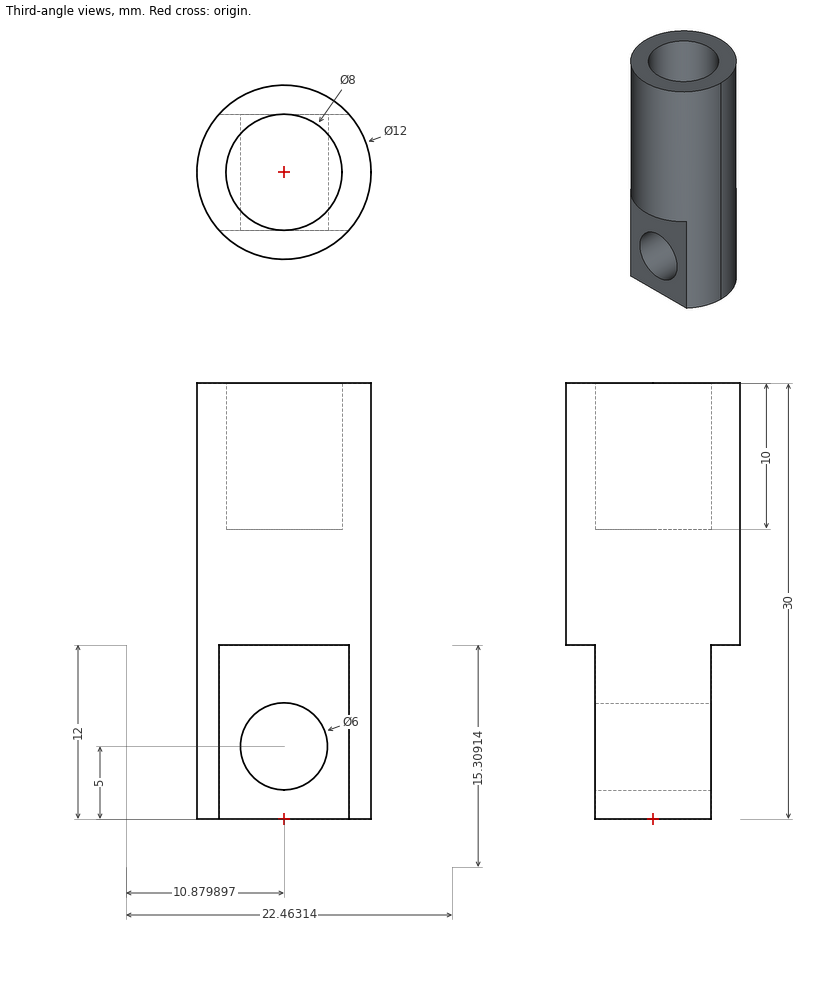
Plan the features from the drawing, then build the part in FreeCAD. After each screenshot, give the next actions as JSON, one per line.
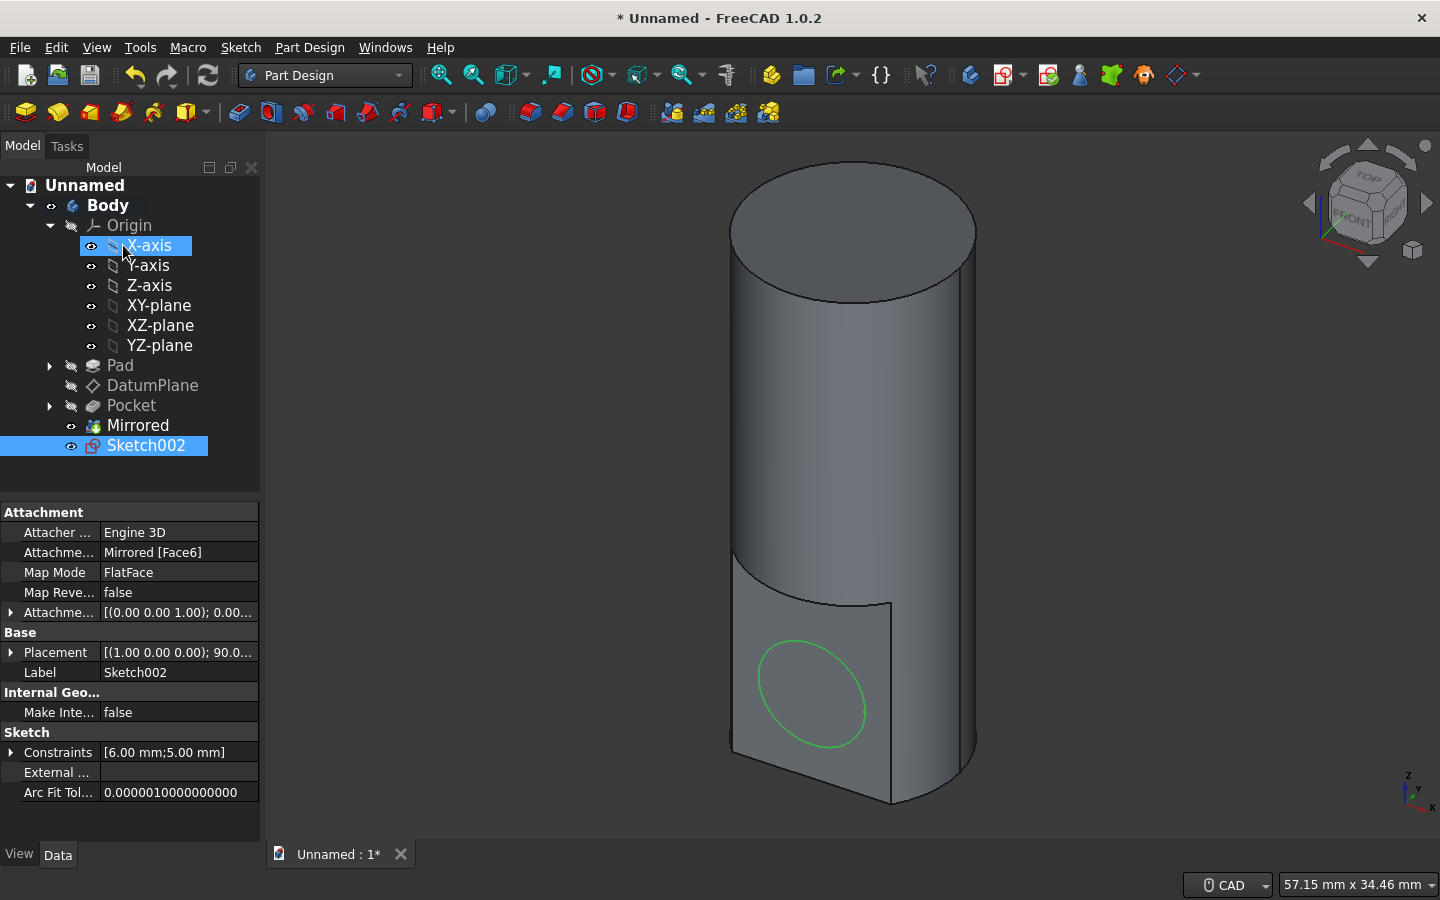
{"action": "left_click", "coordinate": [240, 112]}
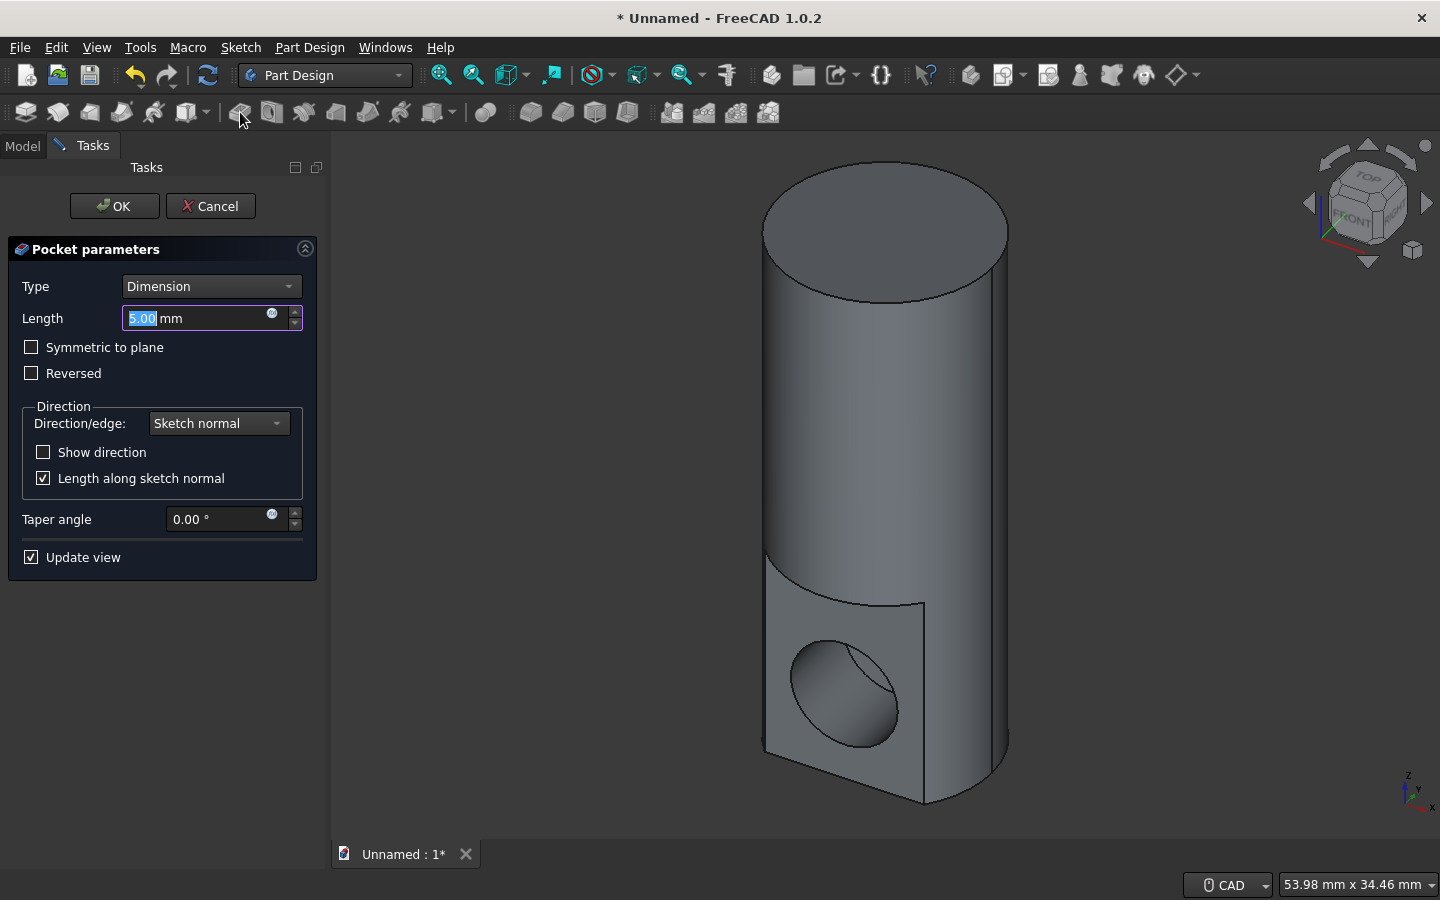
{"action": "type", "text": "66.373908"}
{"action": "key", "text": "Tab"}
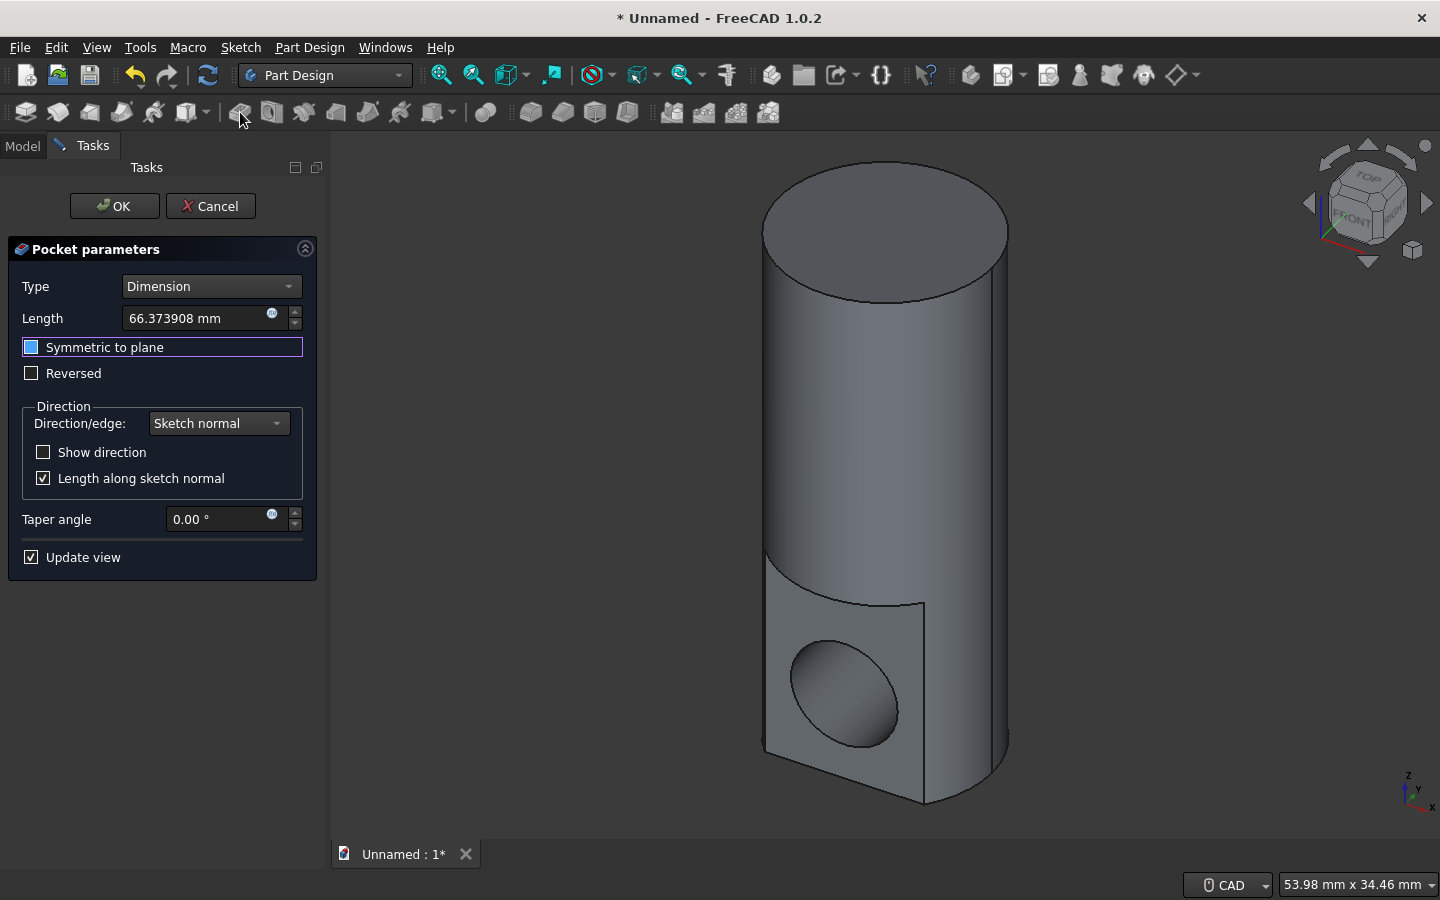
{"action": "left_click", "coordinate": [30, 347]}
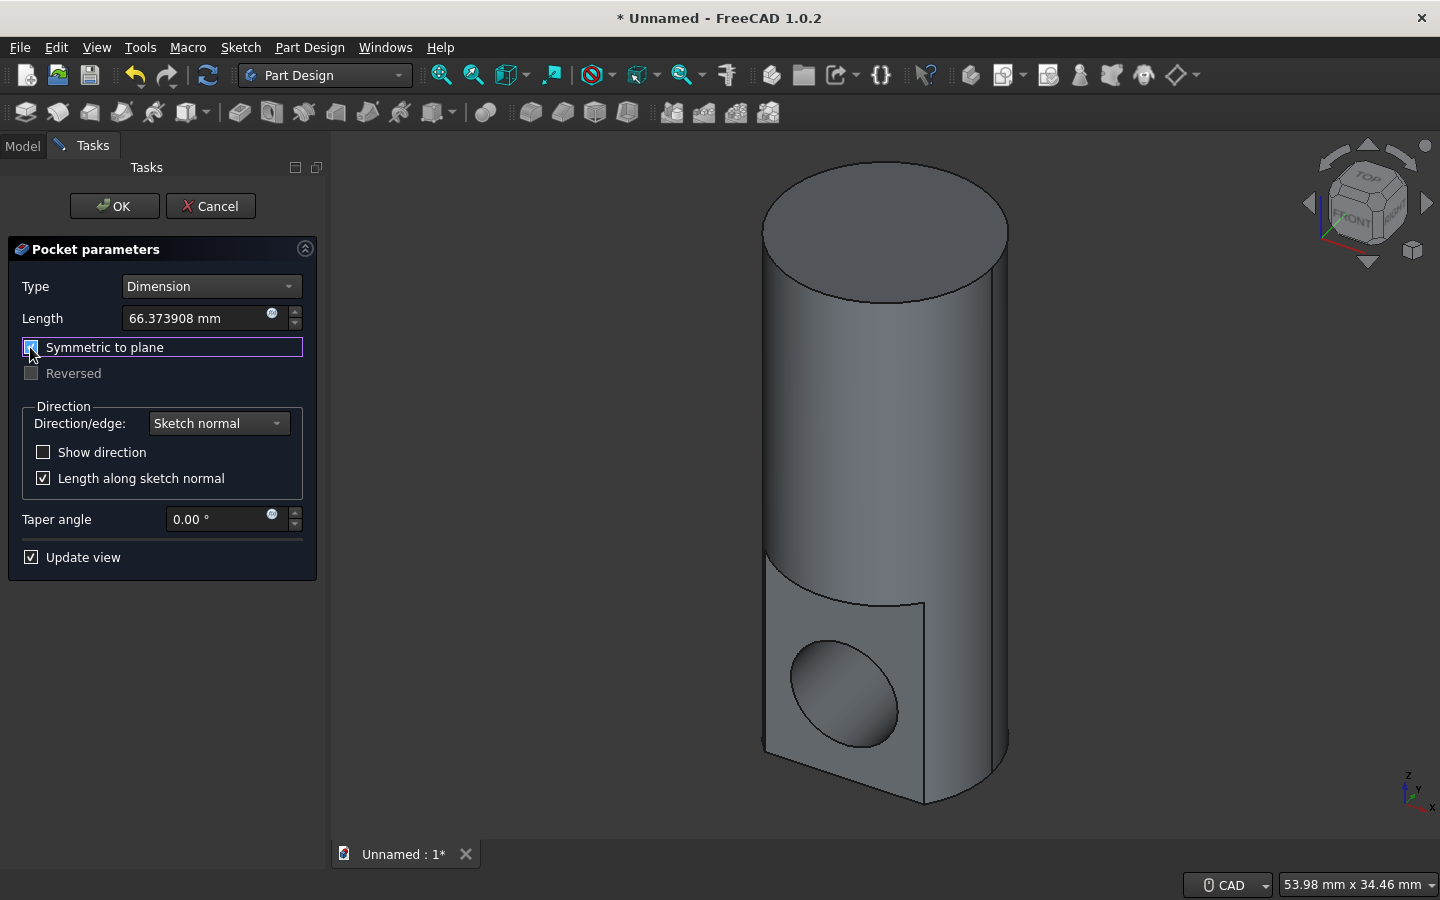
{"action": "left_click", "coordinate": [115, 206]}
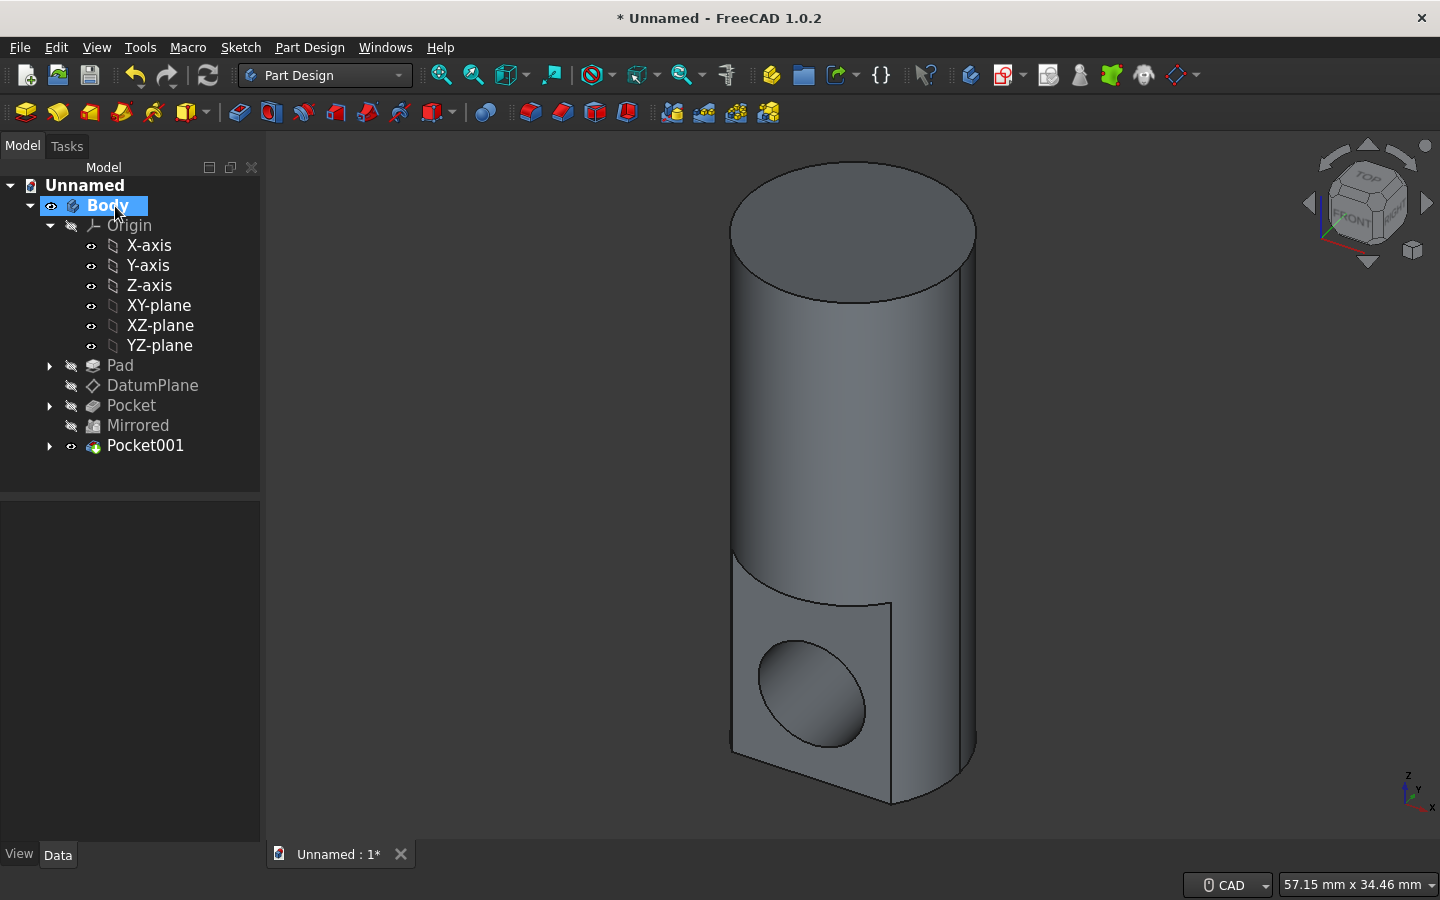
{"action": "left_click", "coordinate": [853, 232]}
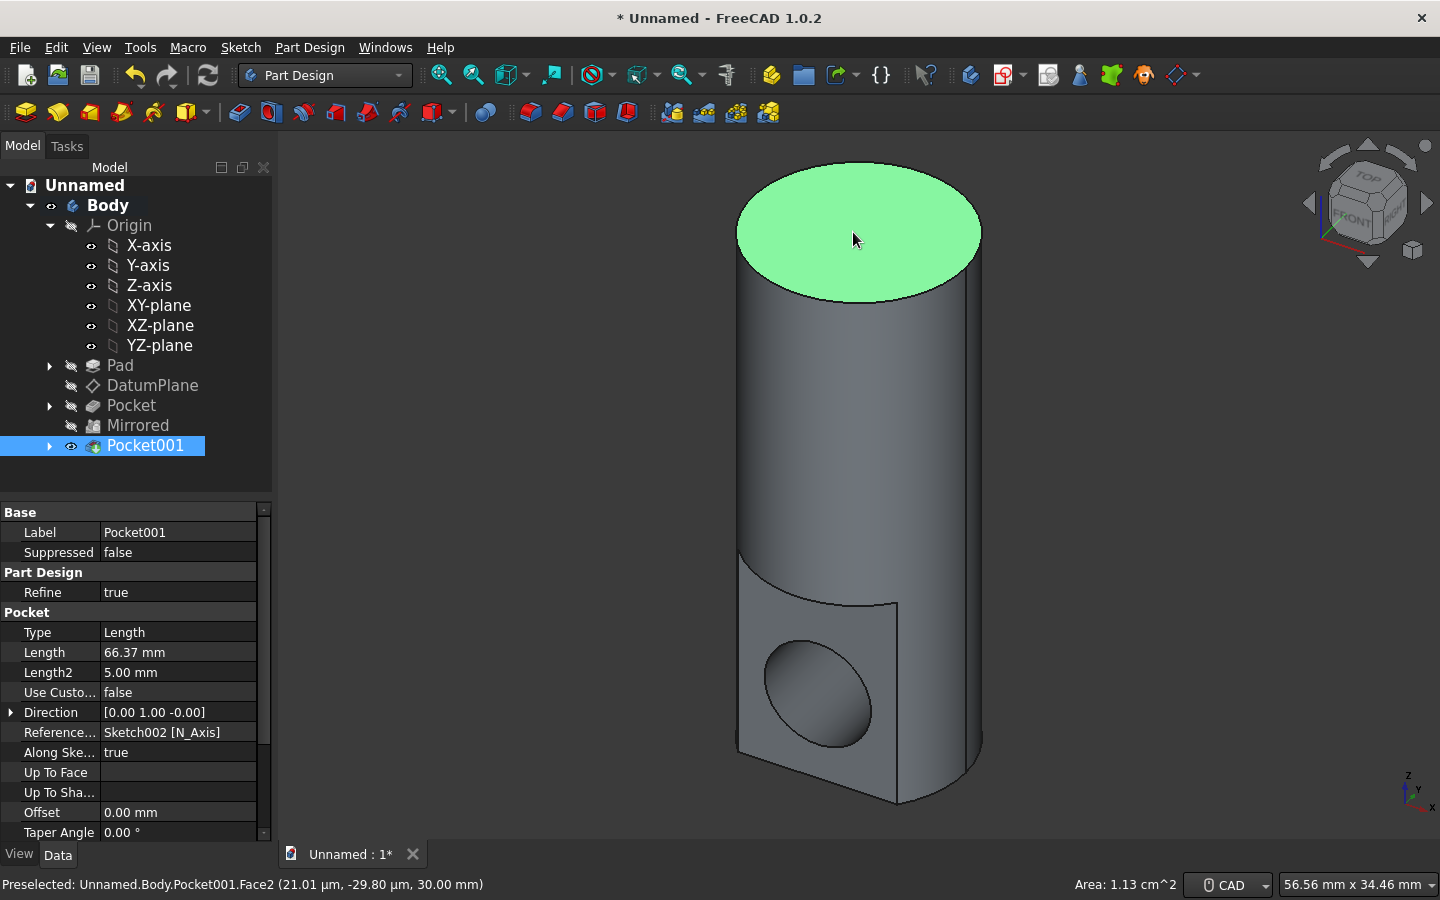
{"action": "left_click", "coordinate": [1004, 76]}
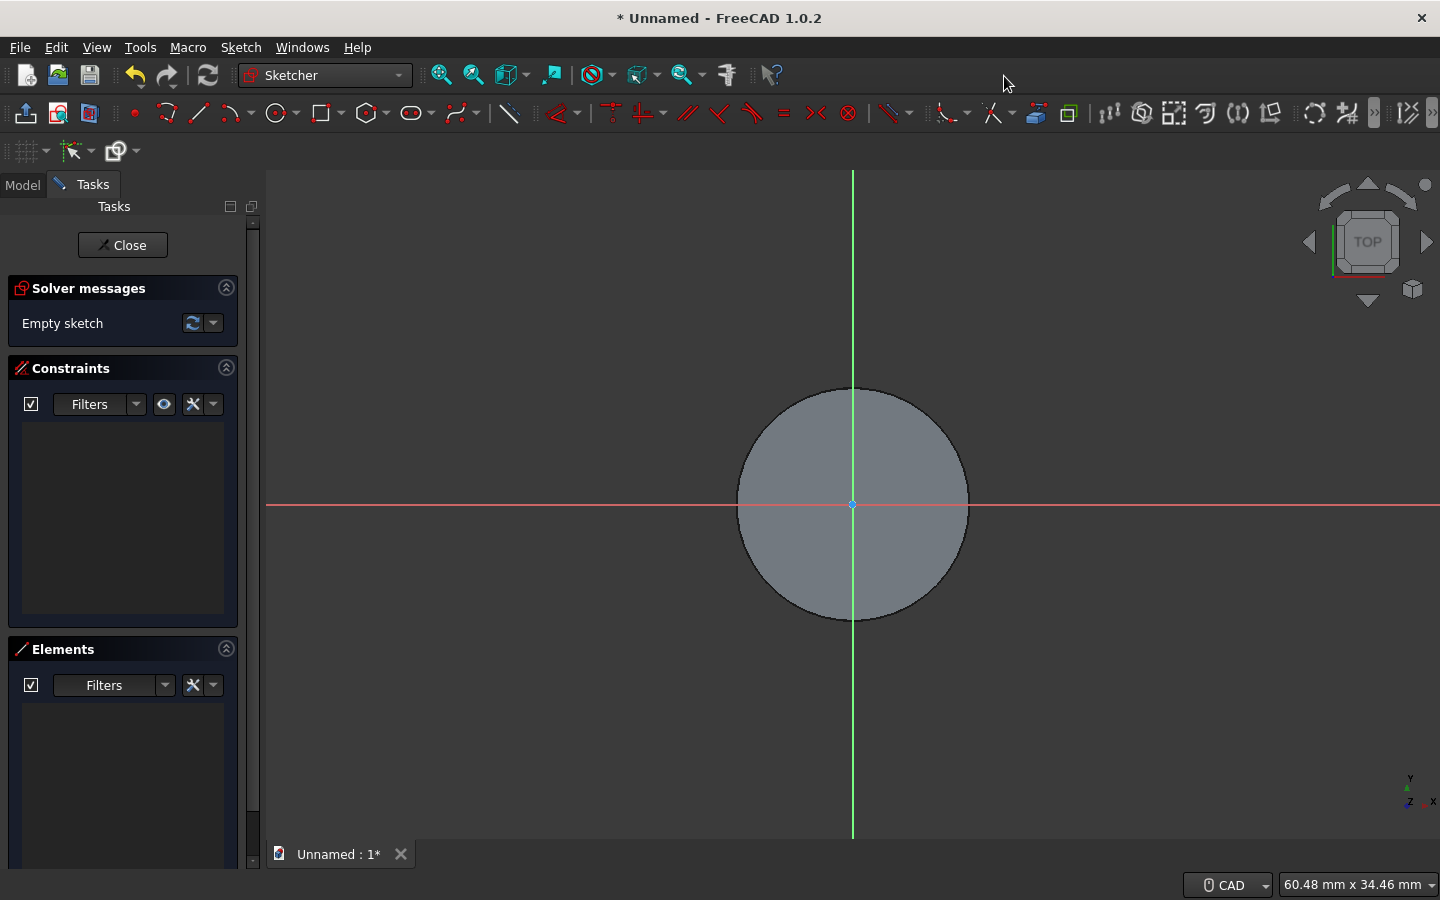
{"action": "scroll", "coordinate": [893, 505], "scroll_direction": "up", "scroll_amount": 5}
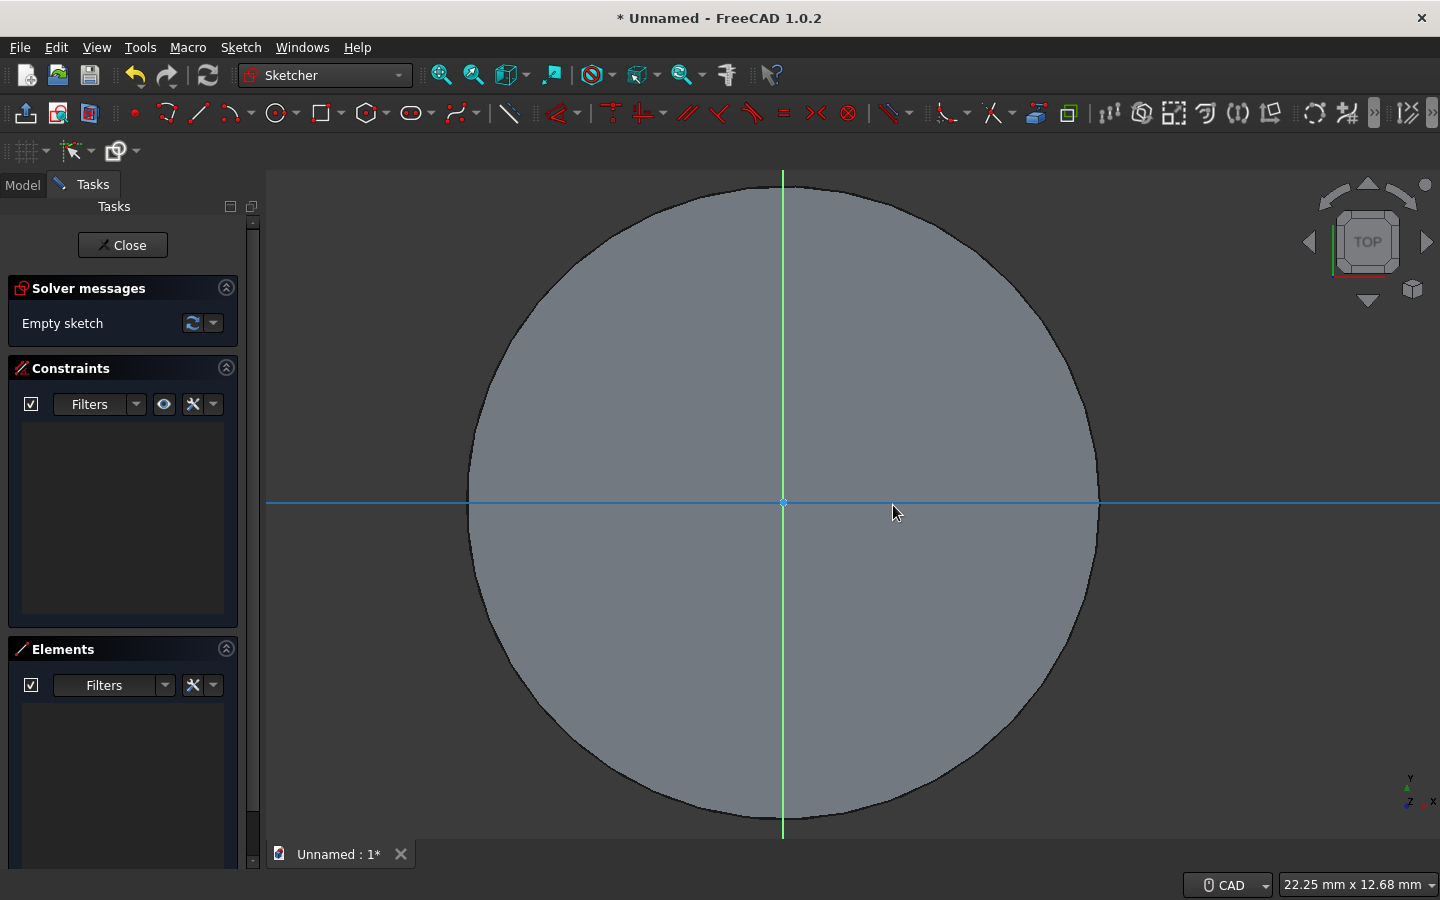
{"action": "left_click", "coordinate": [276, 114]}